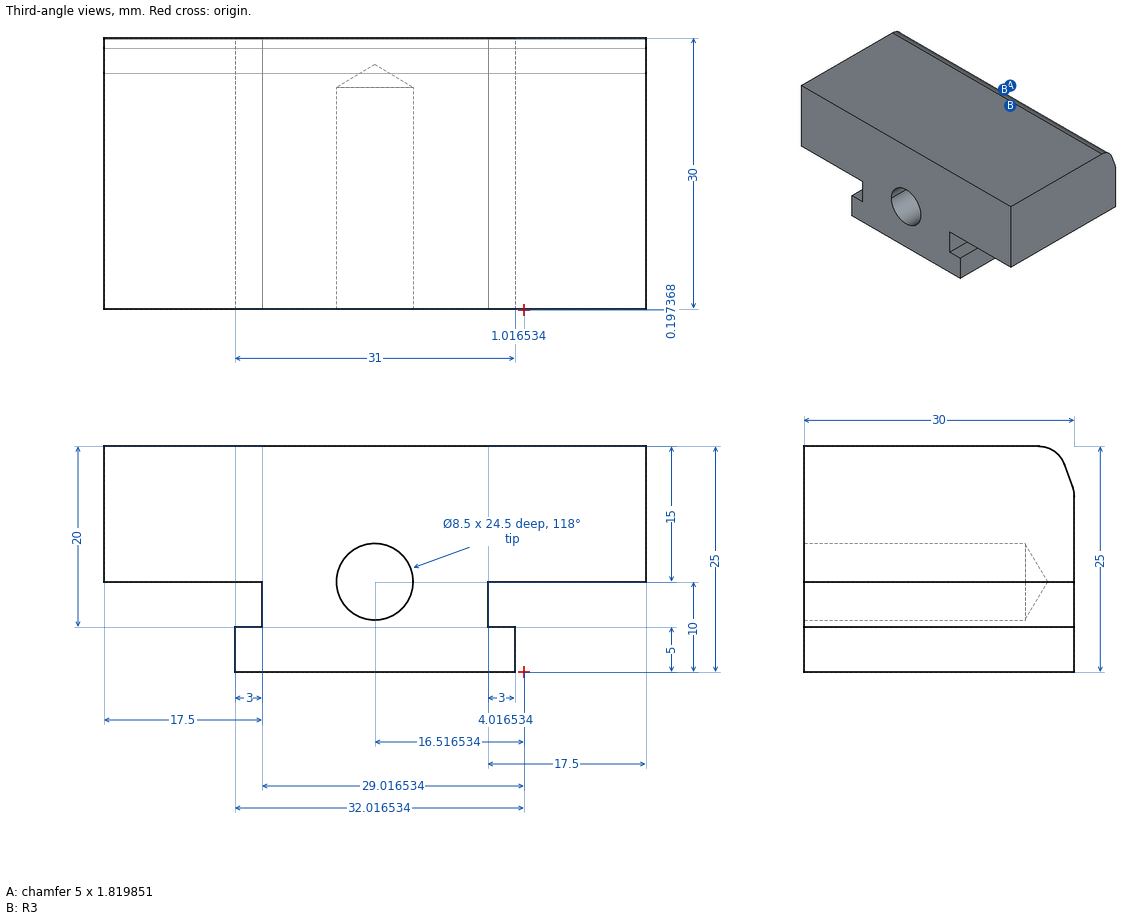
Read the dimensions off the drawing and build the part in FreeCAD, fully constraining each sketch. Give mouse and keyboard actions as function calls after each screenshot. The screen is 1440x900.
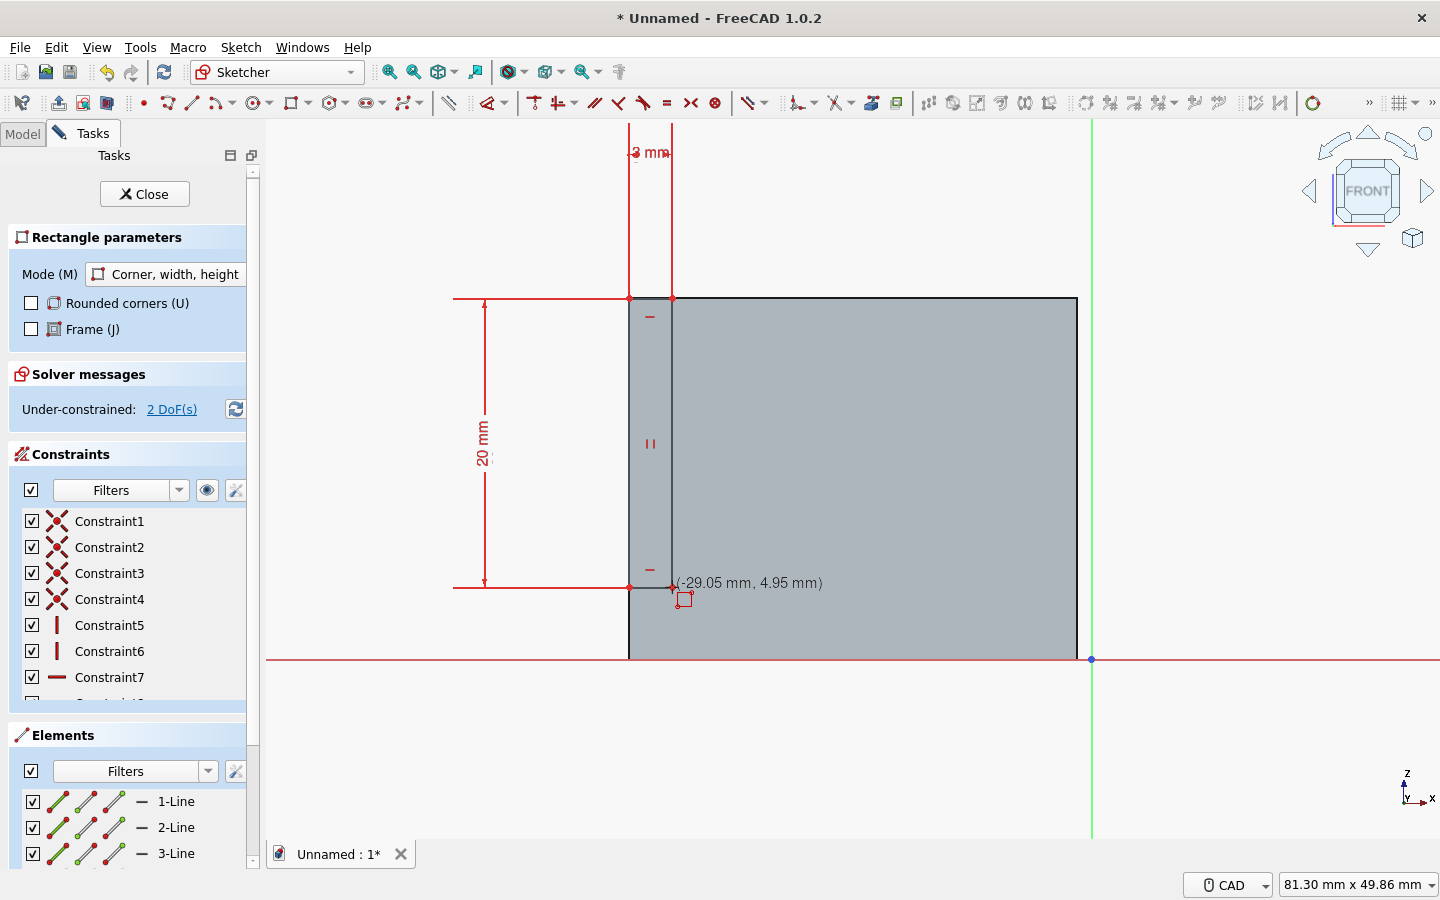
click(1034, 298)
move(1077, 587)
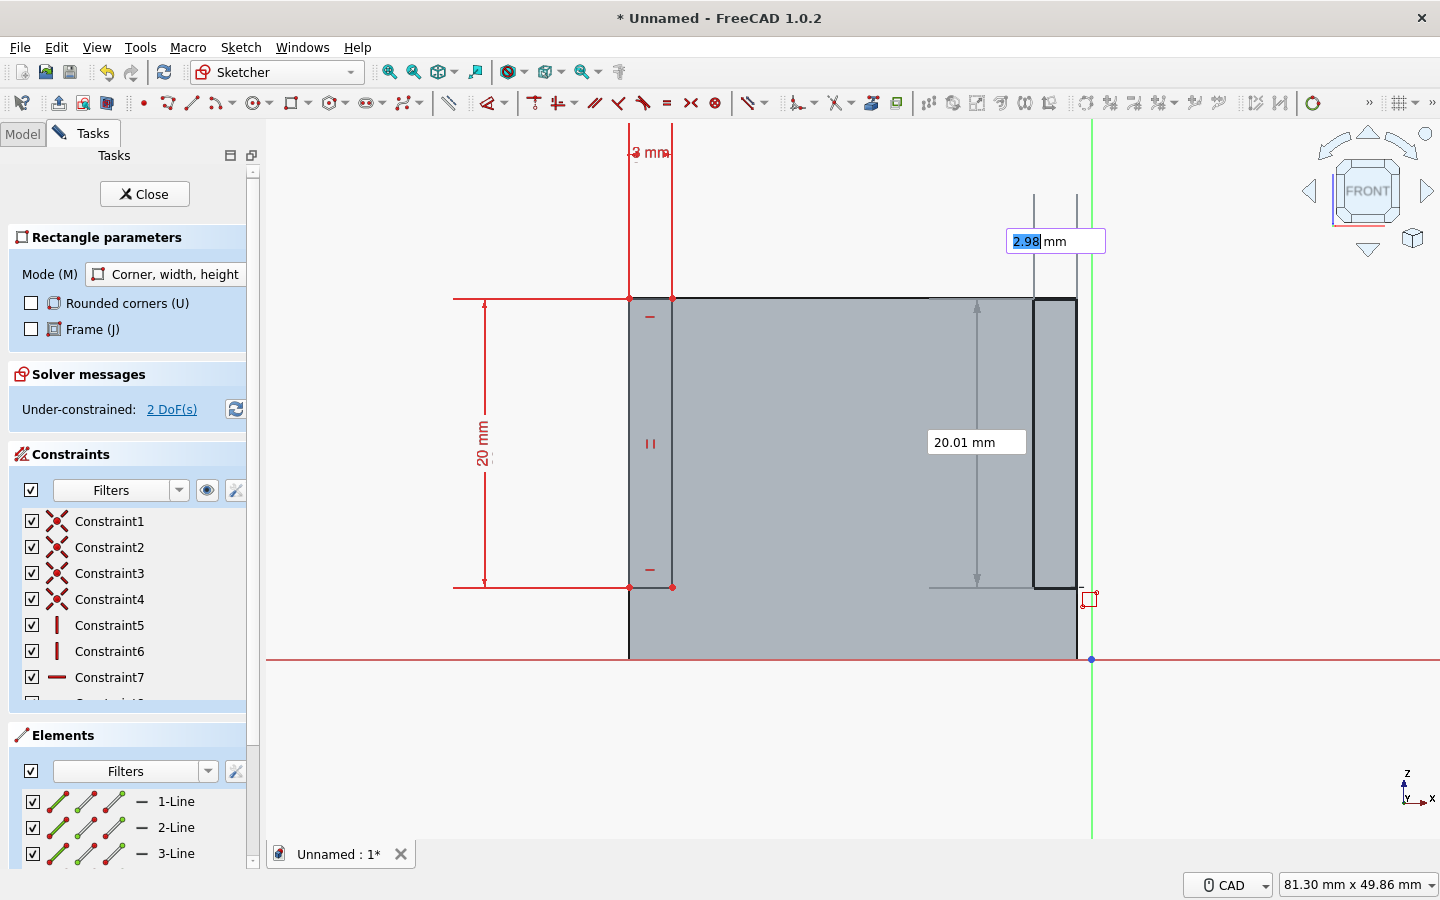
text(3)
key(Tab)
text(20)
key(Return)
key(Escape)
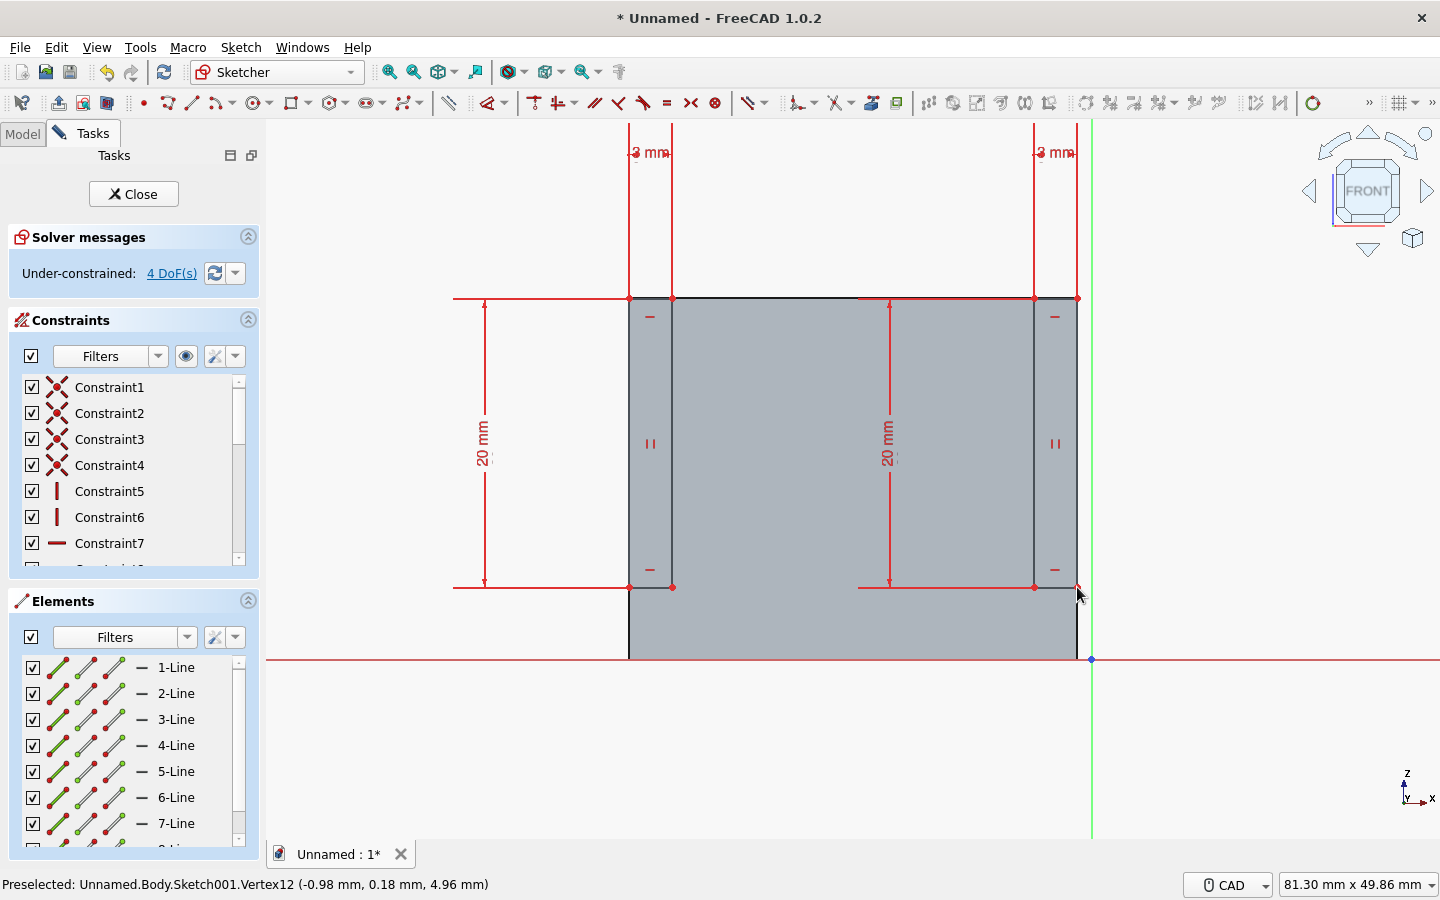
click(488, 104)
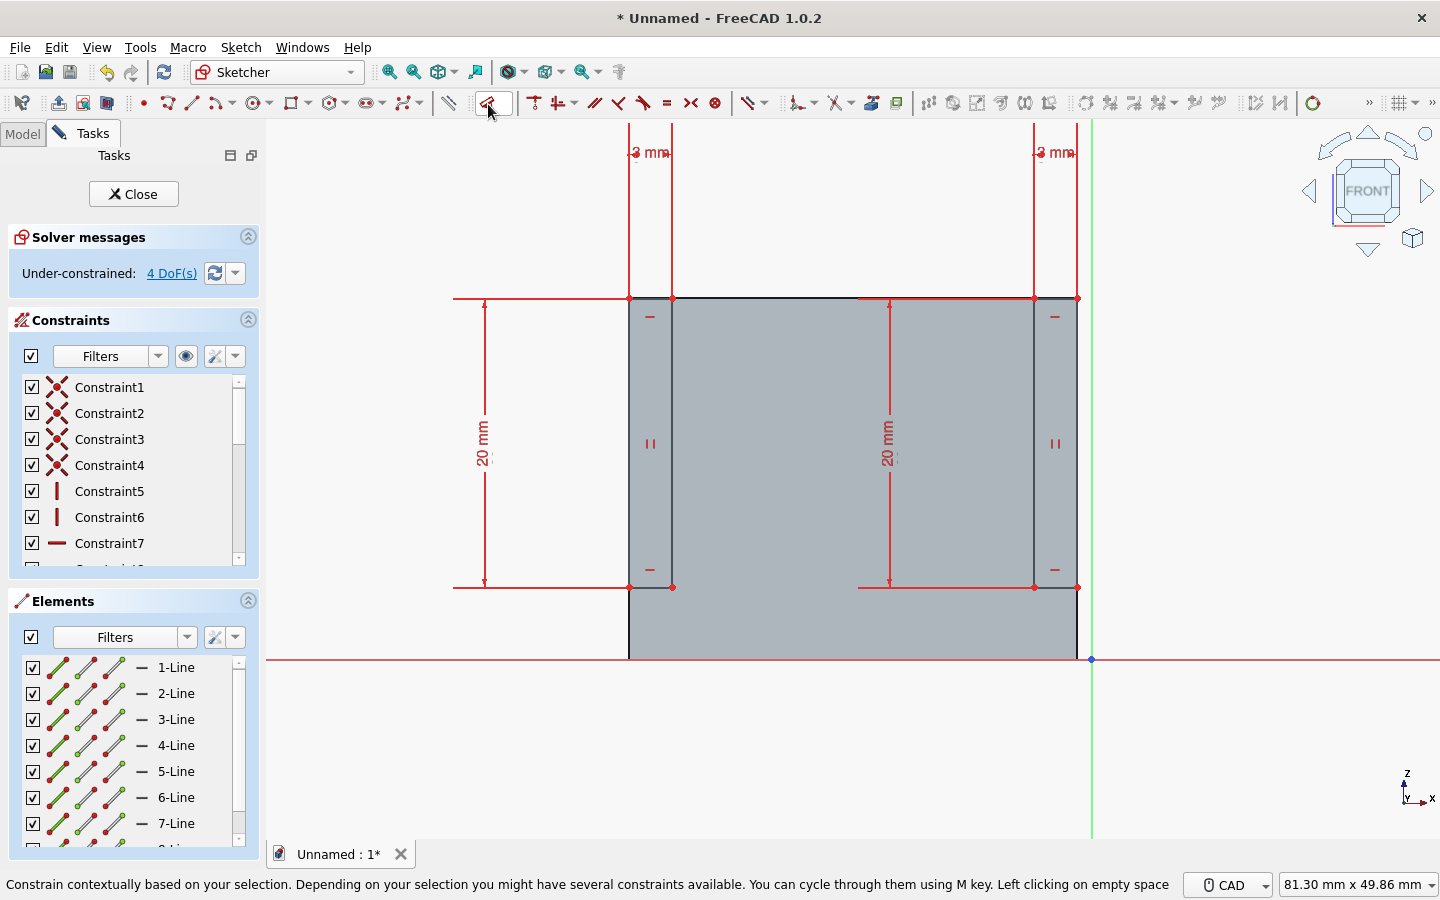
click(629, 588)
click(595, 624)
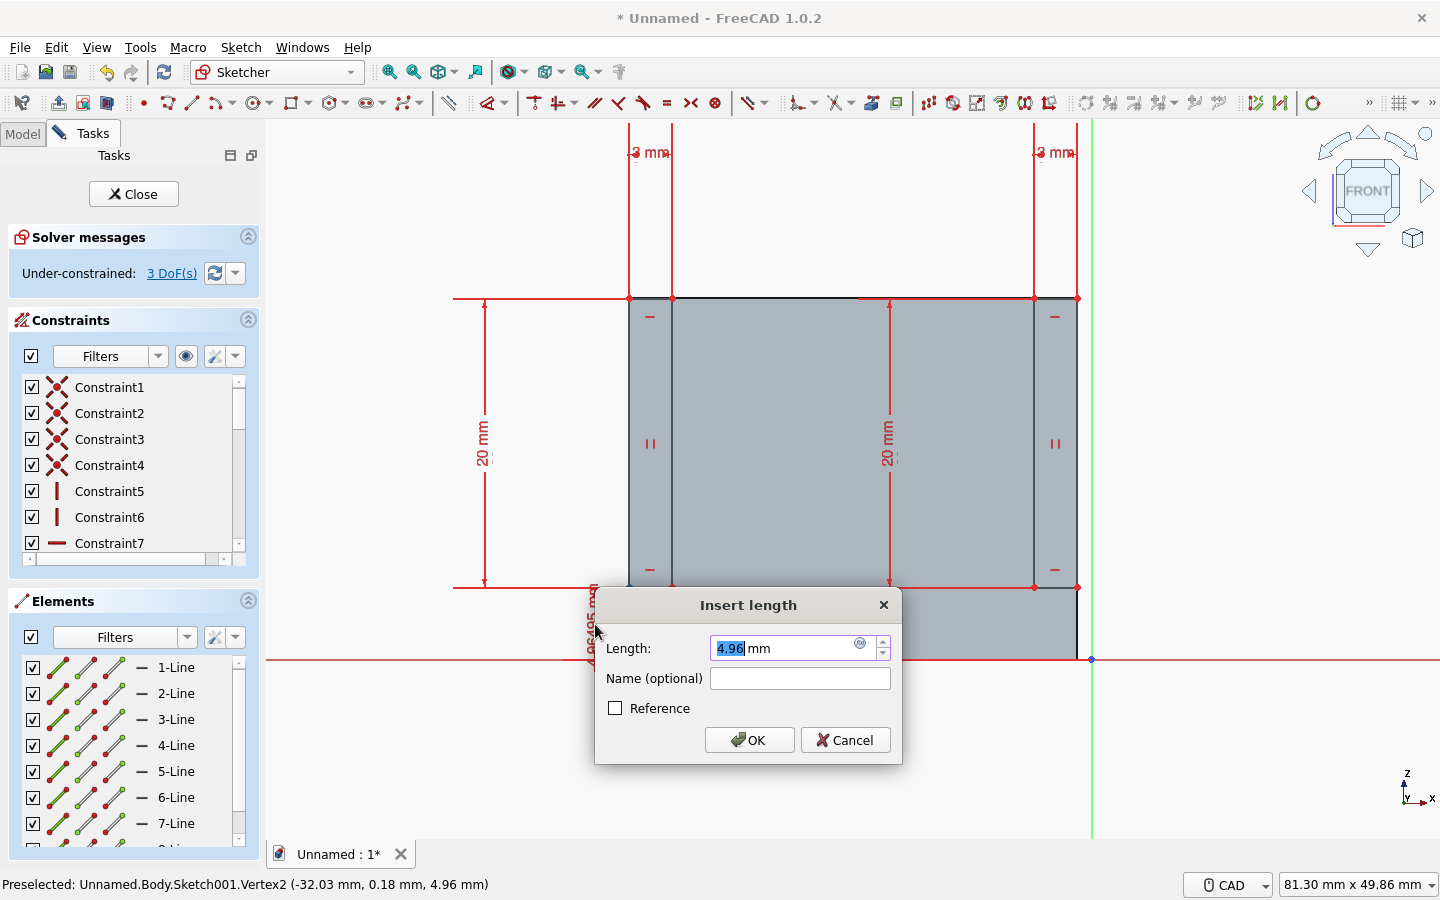
text(5)
key(Return)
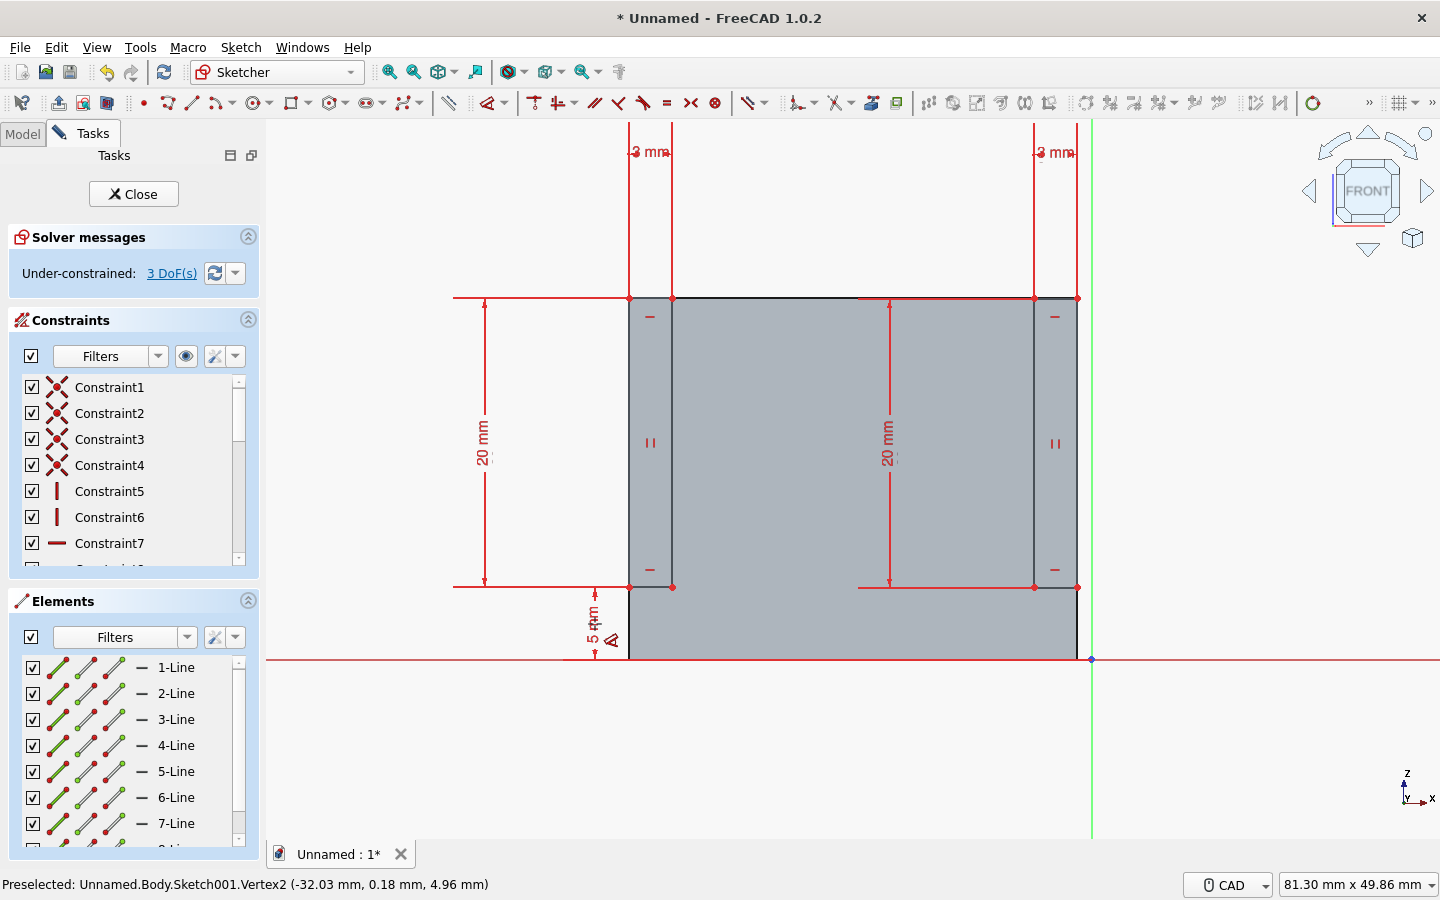
click(1034, 588)
click(1126, 624)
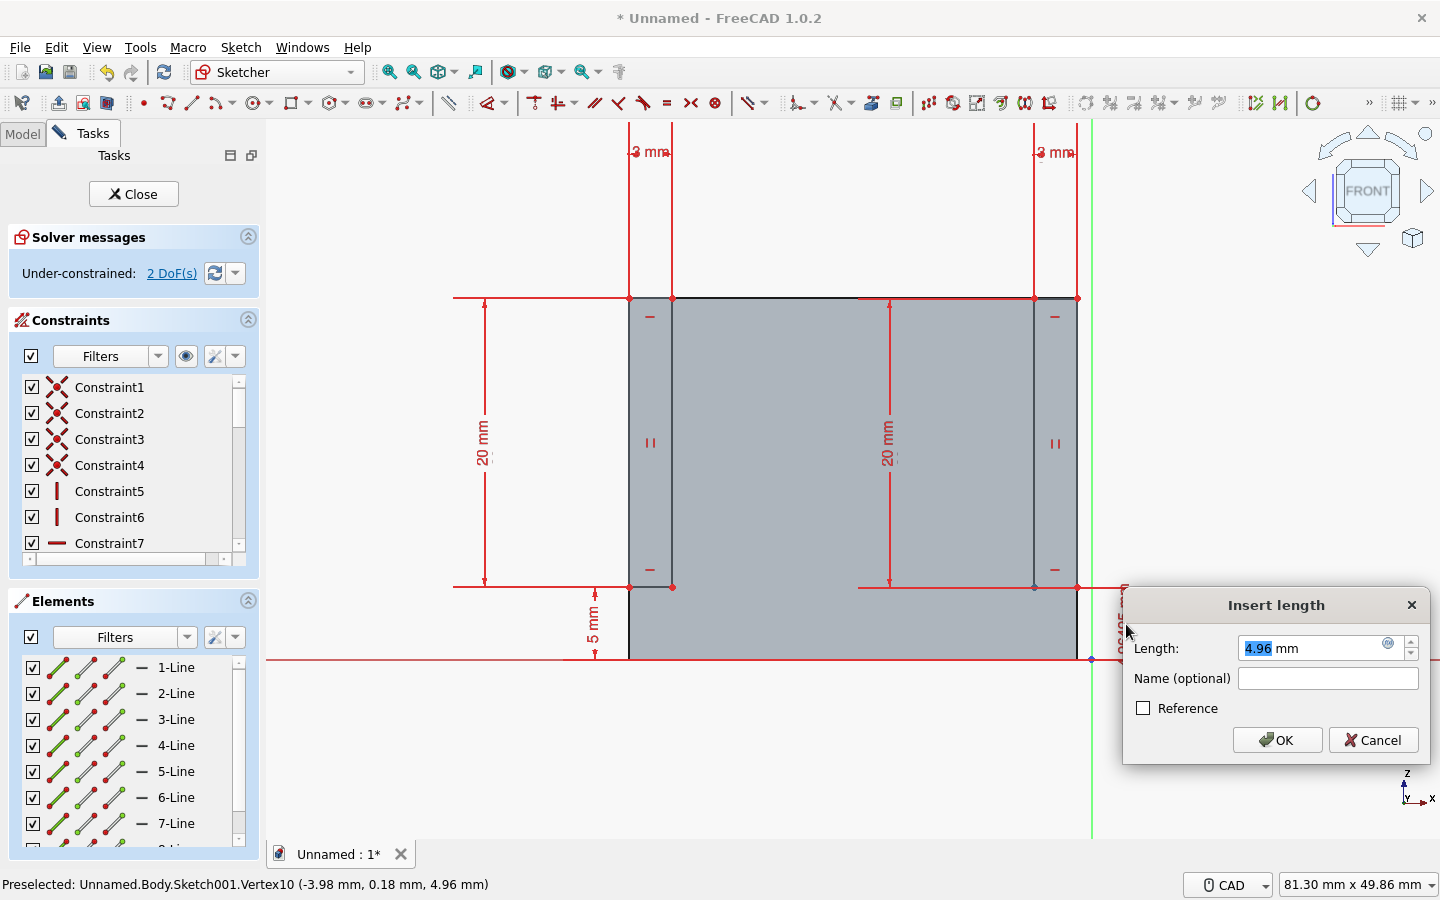
text(5)
key(Return)